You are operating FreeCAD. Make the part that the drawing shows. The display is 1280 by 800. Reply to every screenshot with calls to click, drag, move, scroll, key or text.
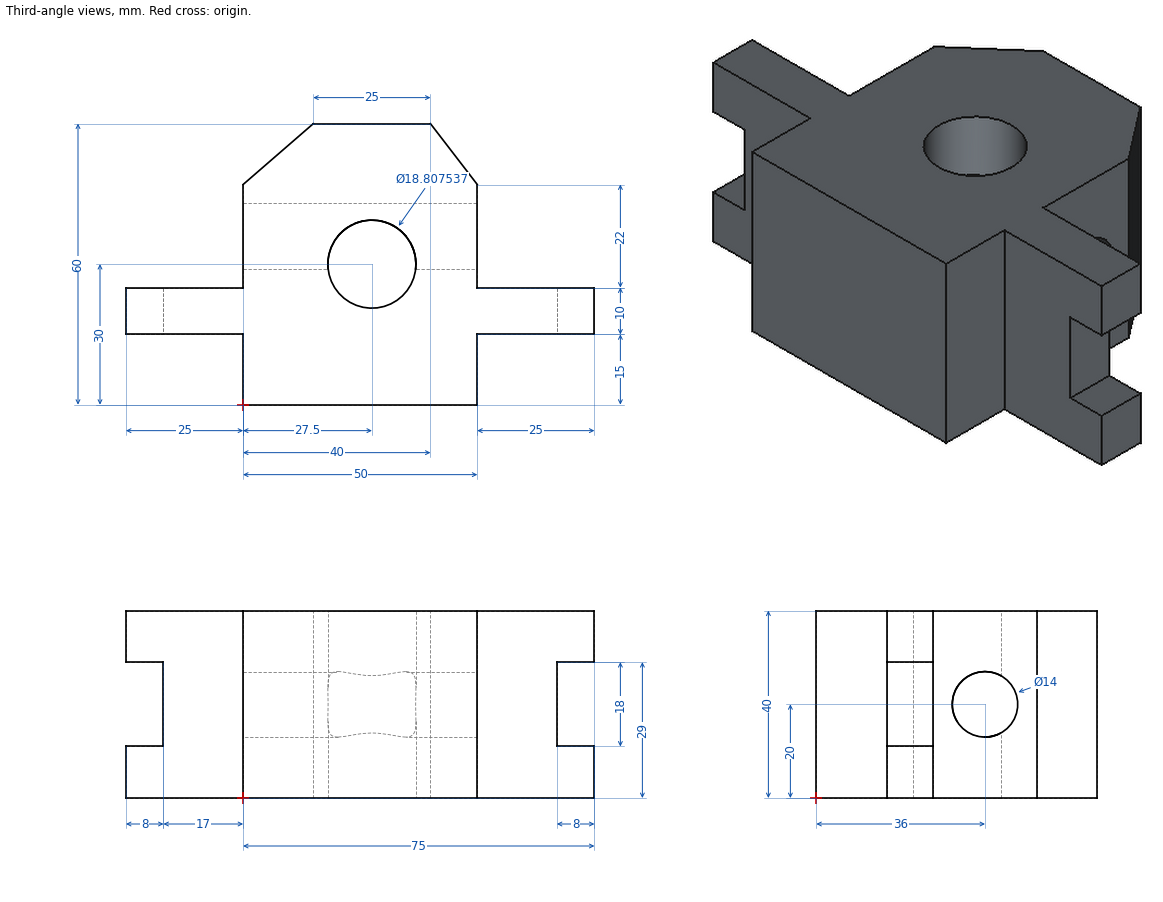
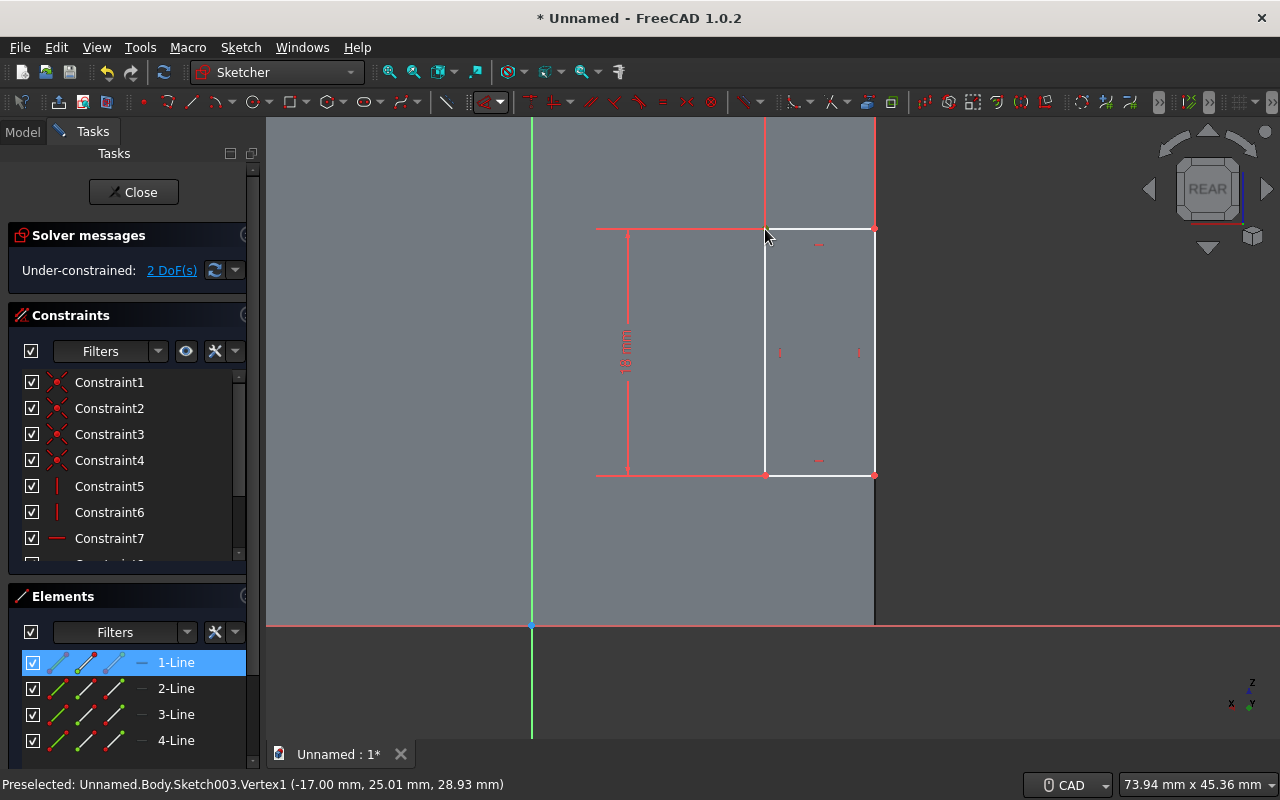
key(l)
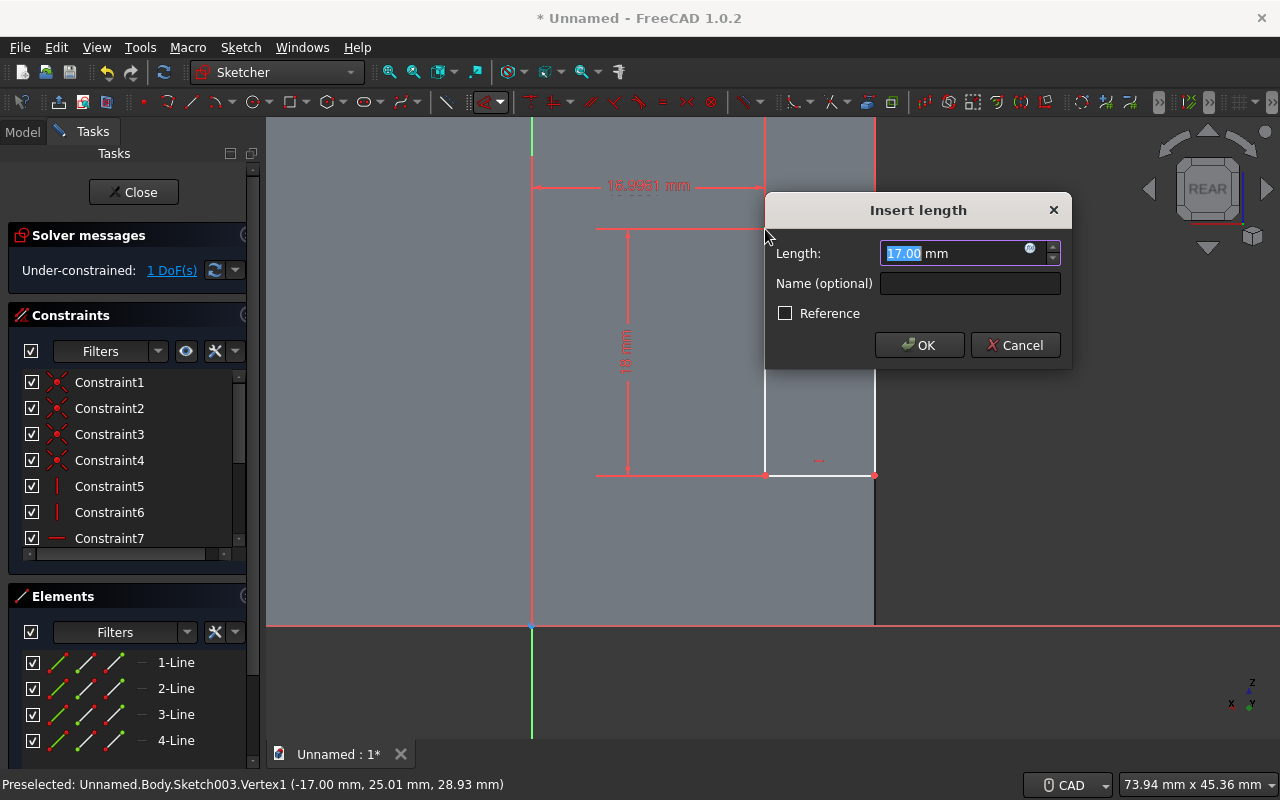
text(17)
key(Return)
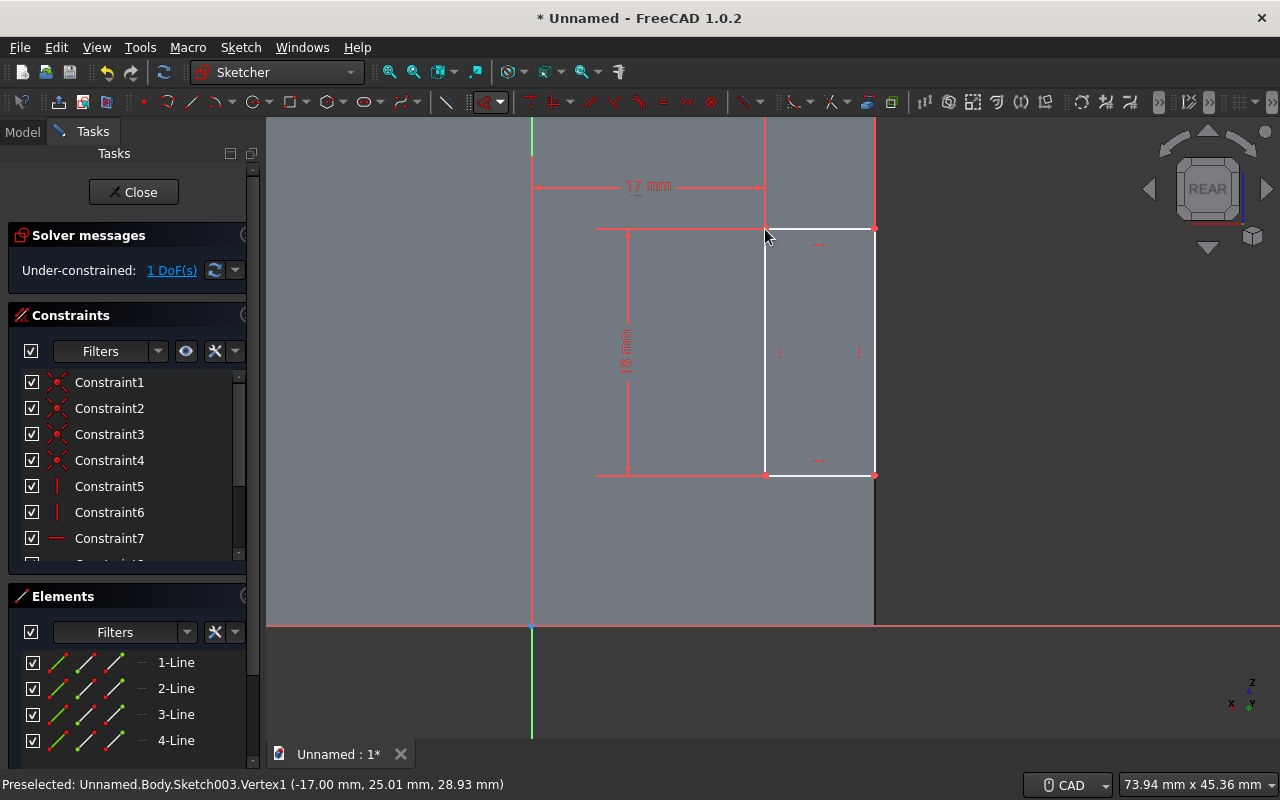
click(765, 229)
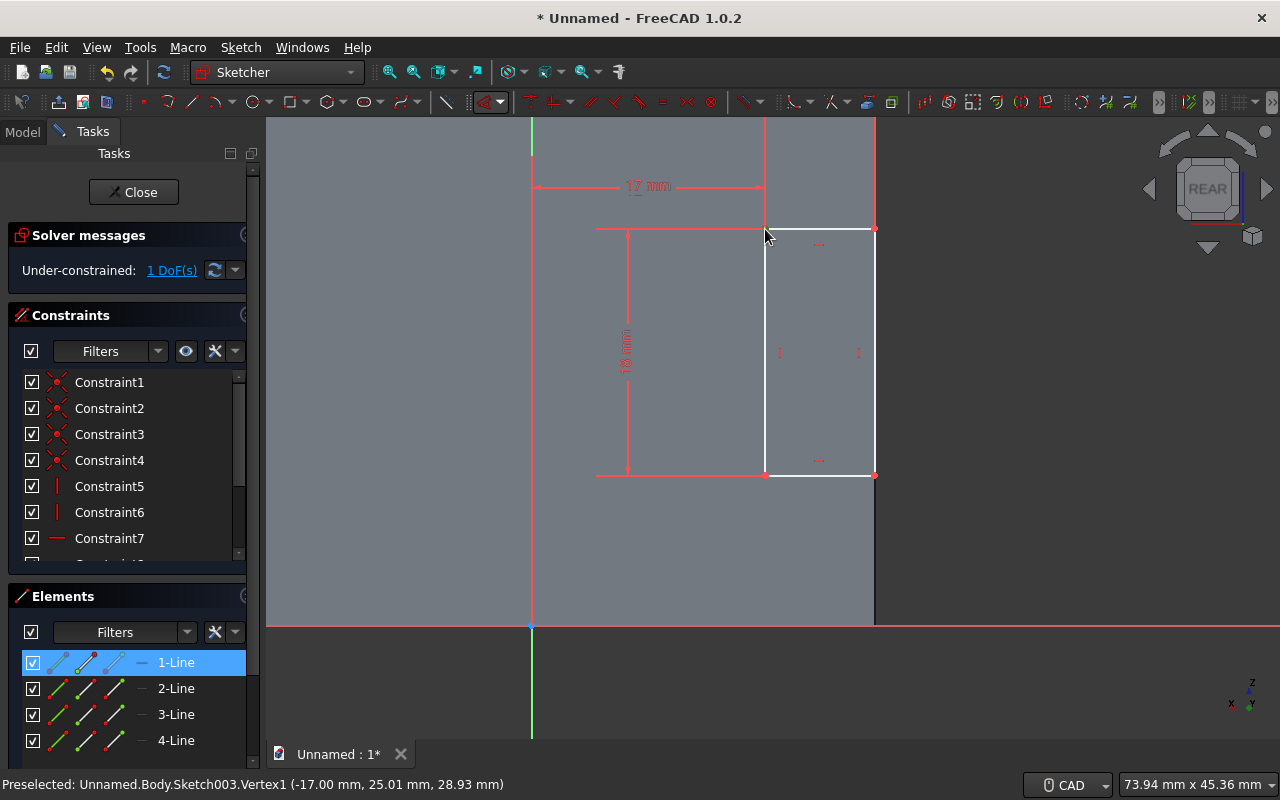
key(i)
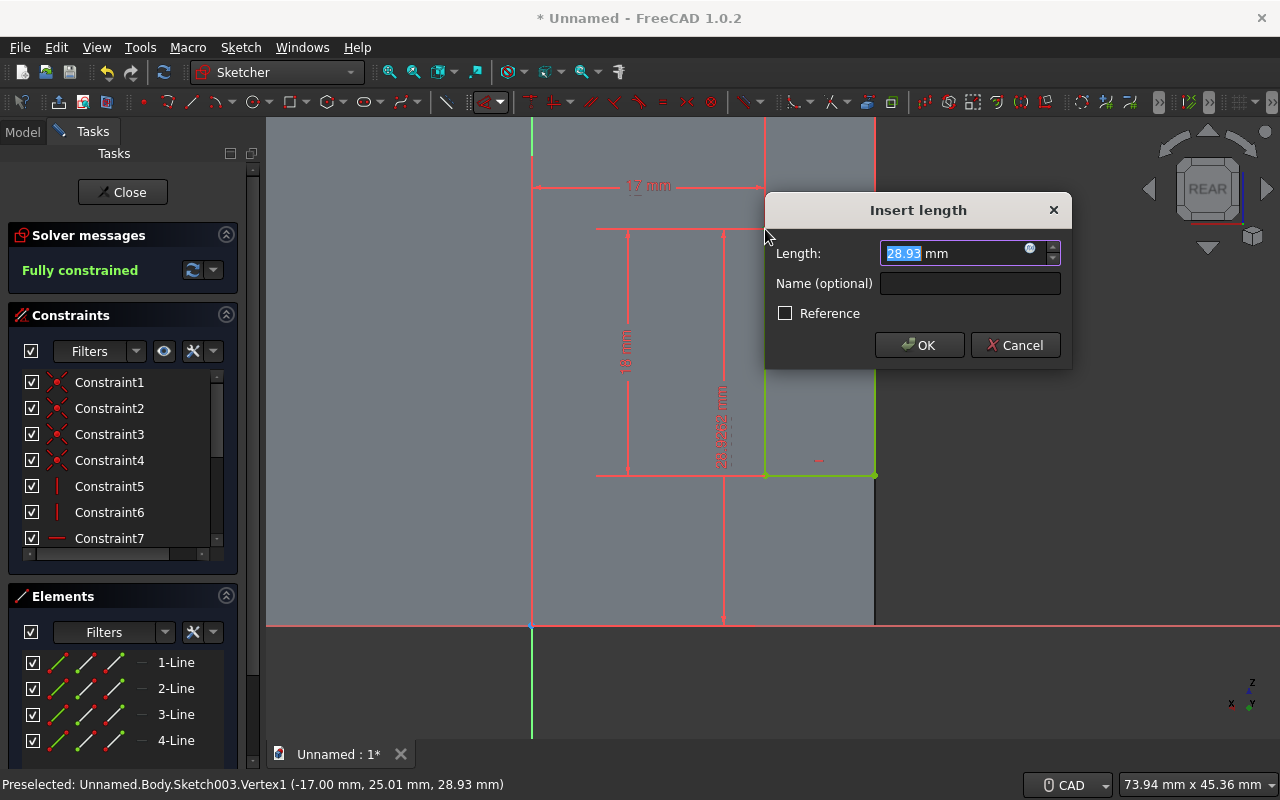
text(29)
key(Return)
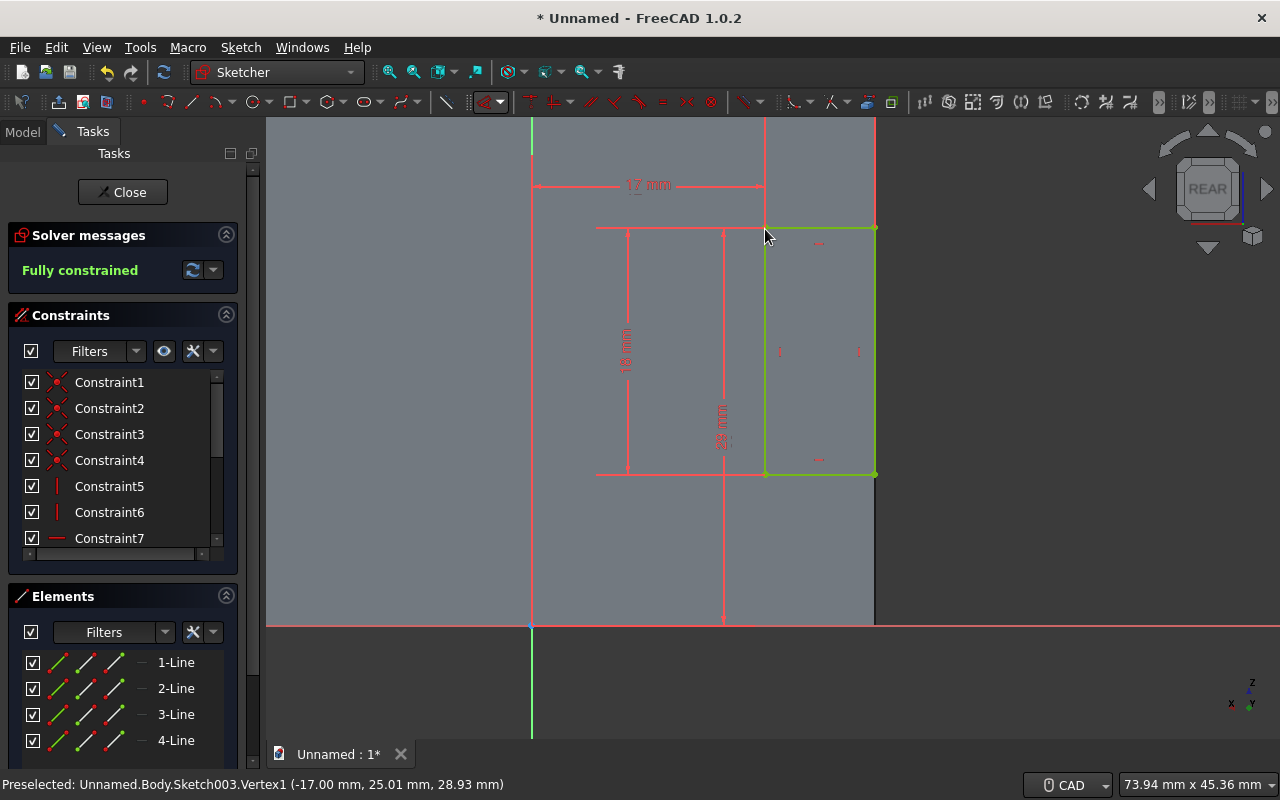
click(123, 192)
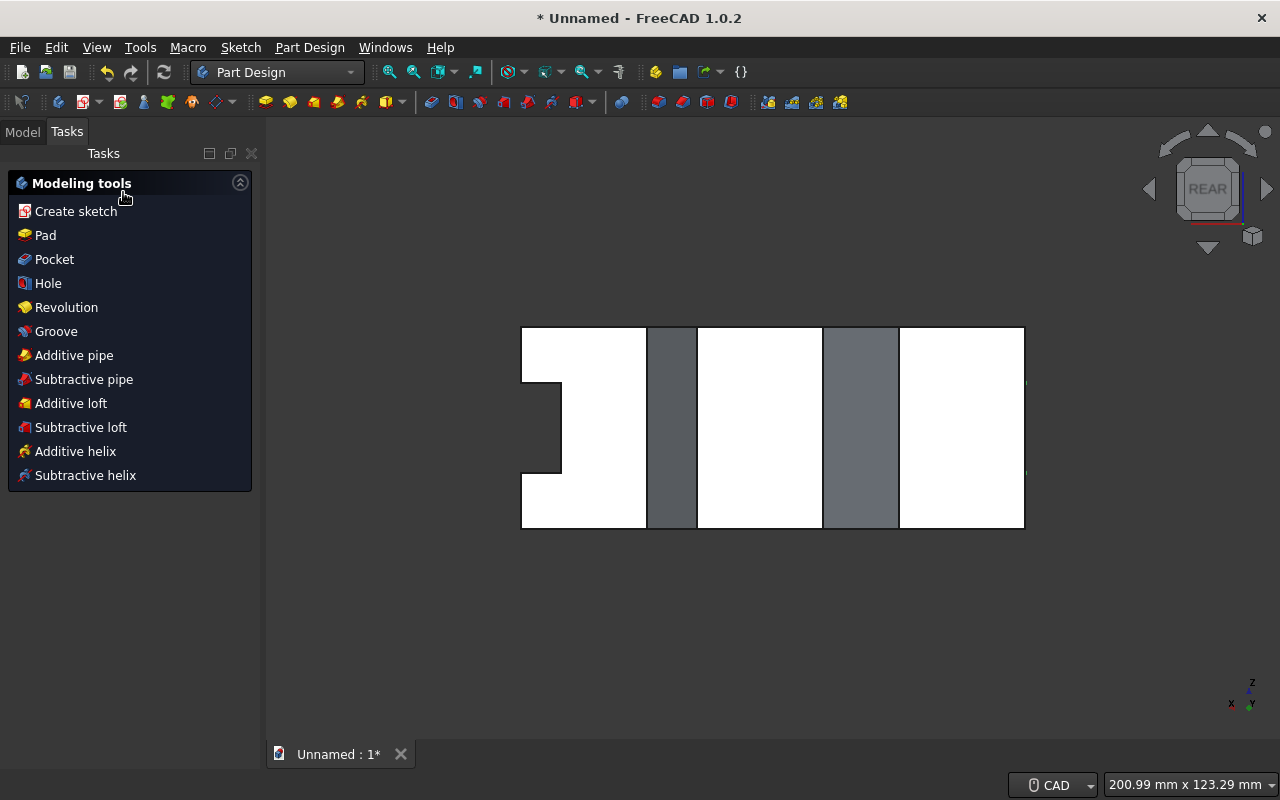
click(432, 102)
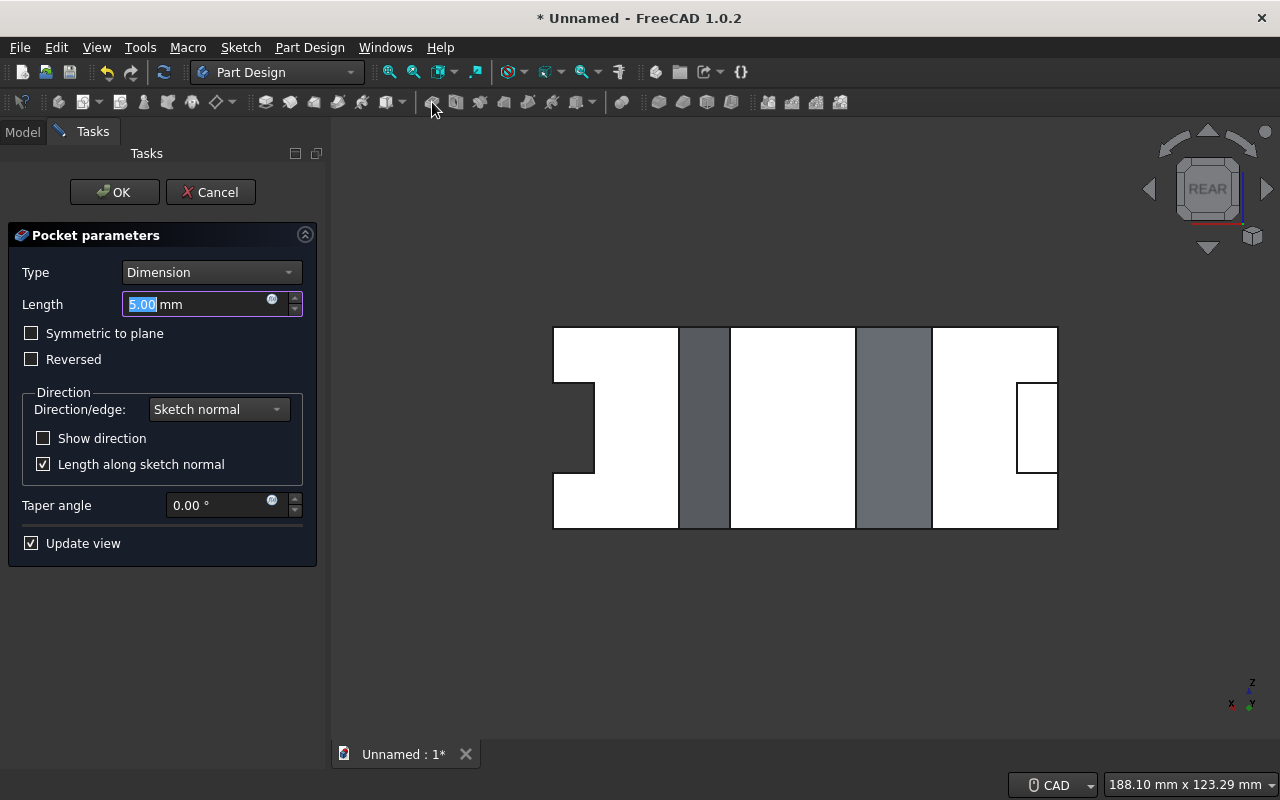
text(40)
key(Tab)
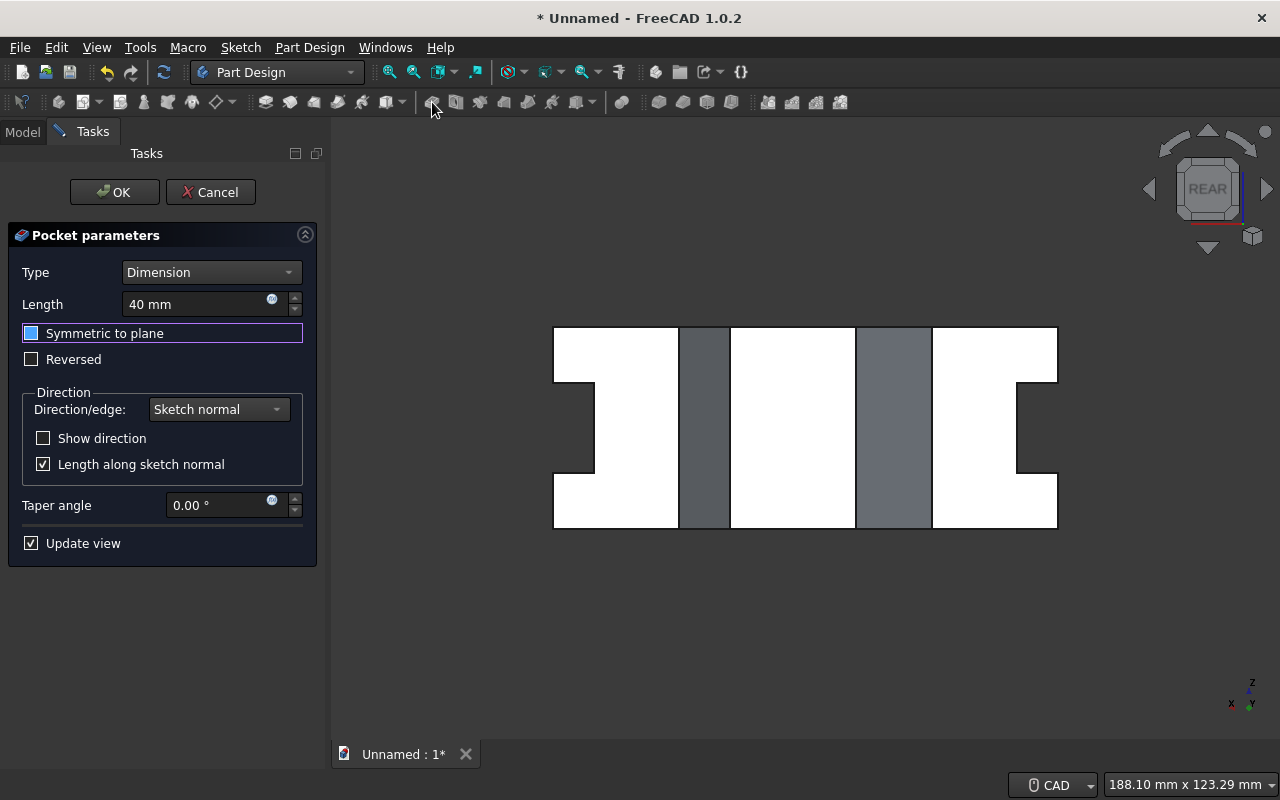
click(115, 192)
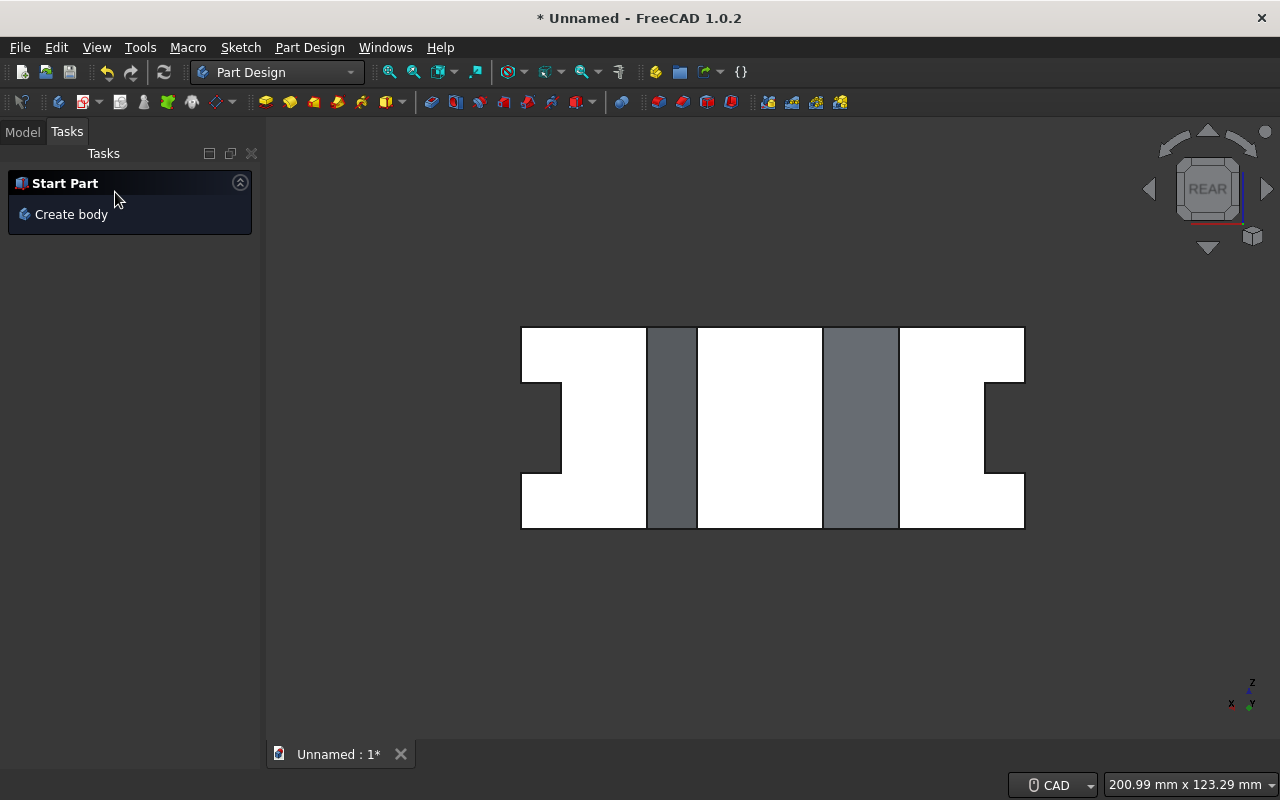
key(0)